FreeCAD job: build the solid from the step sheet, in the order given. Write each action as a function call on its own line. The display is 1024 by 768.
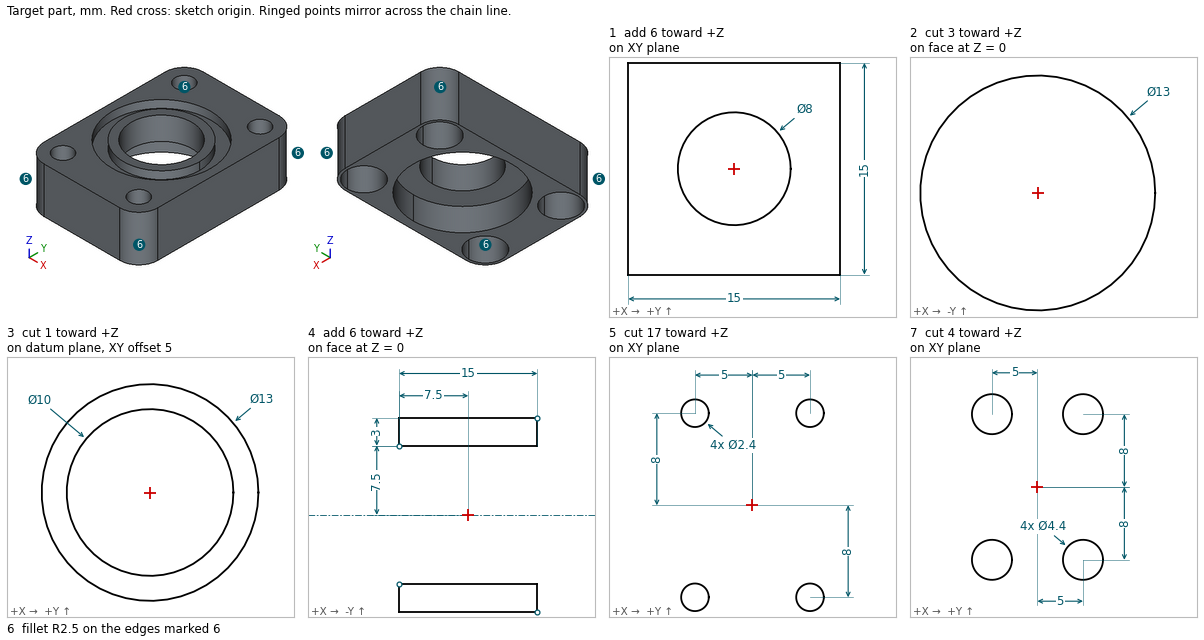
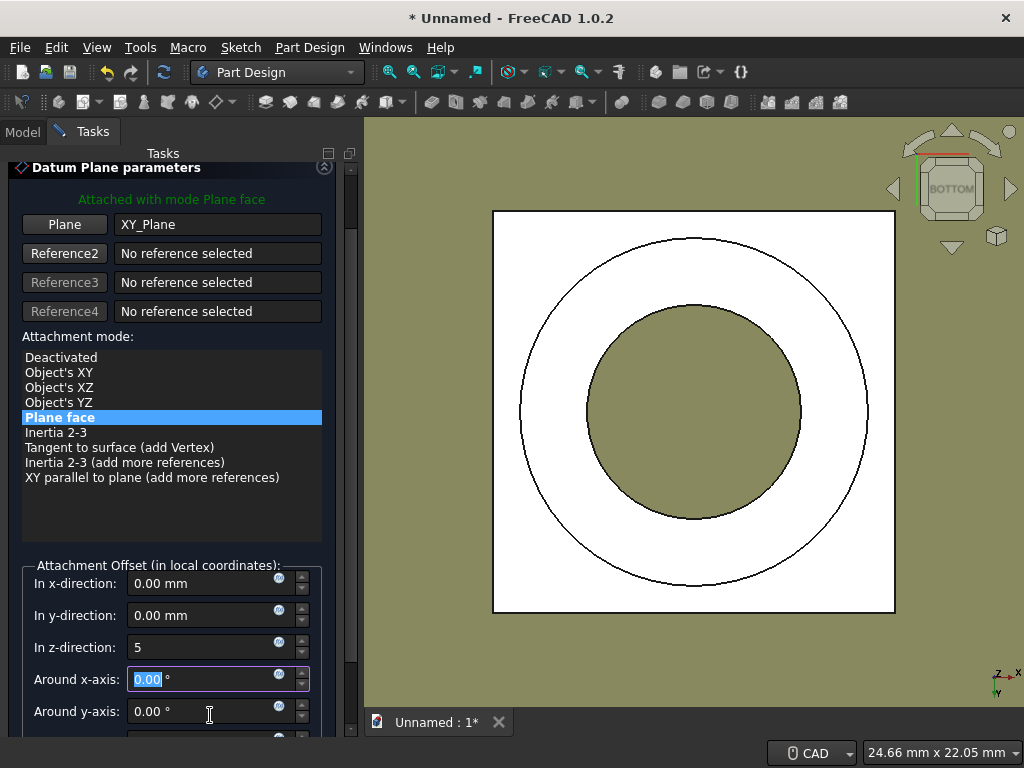
scroll(351, 450, up, 2)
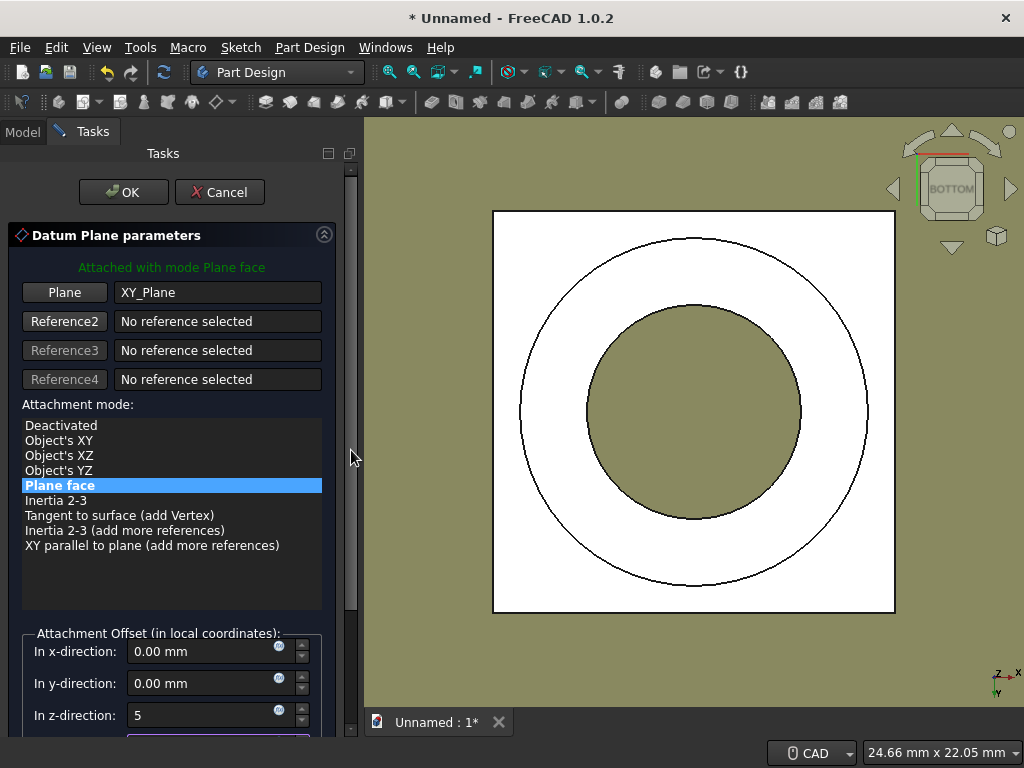
click(124, 192)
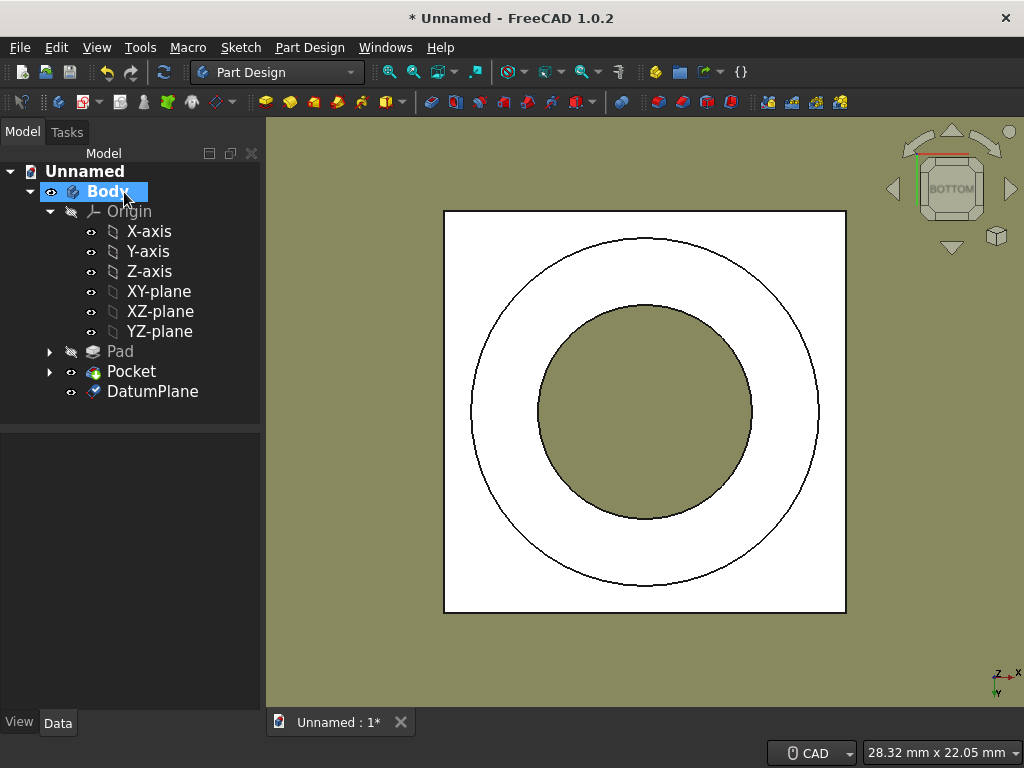
click(116, 392)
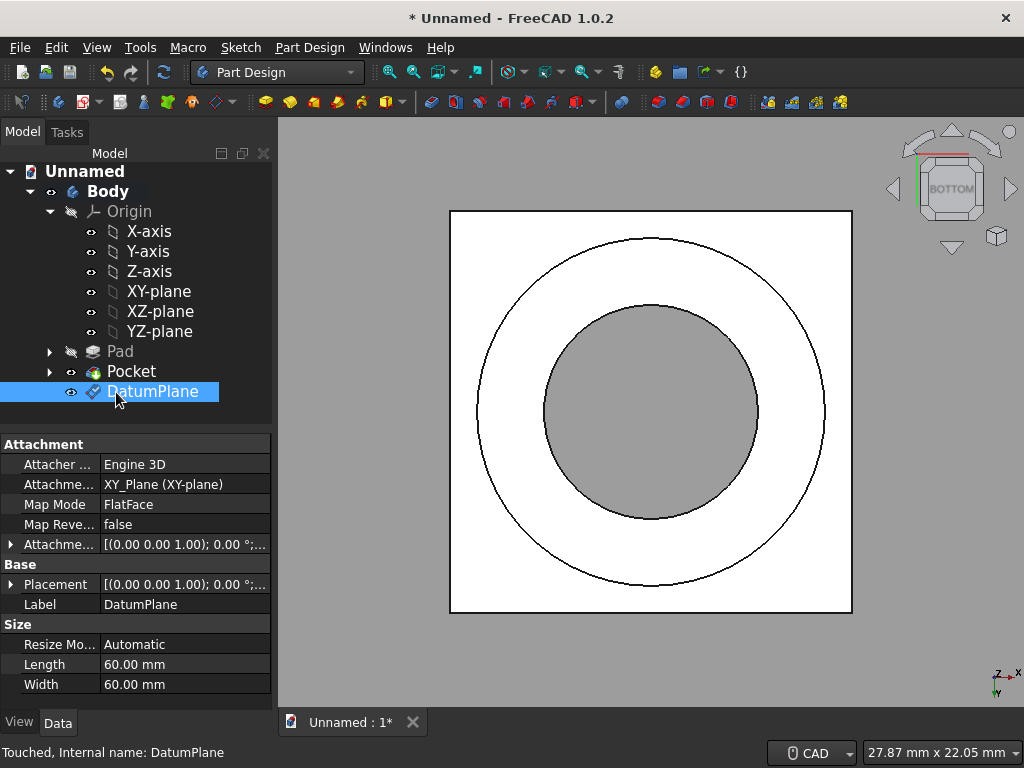
click(84, 102)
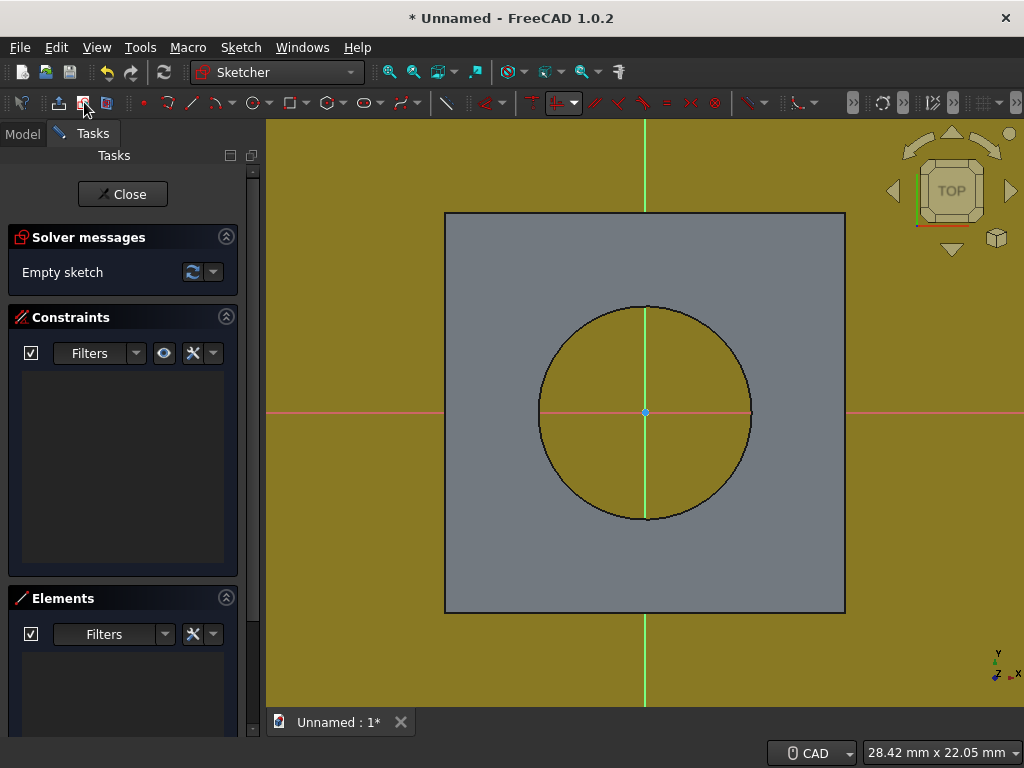
key(q)
key(s)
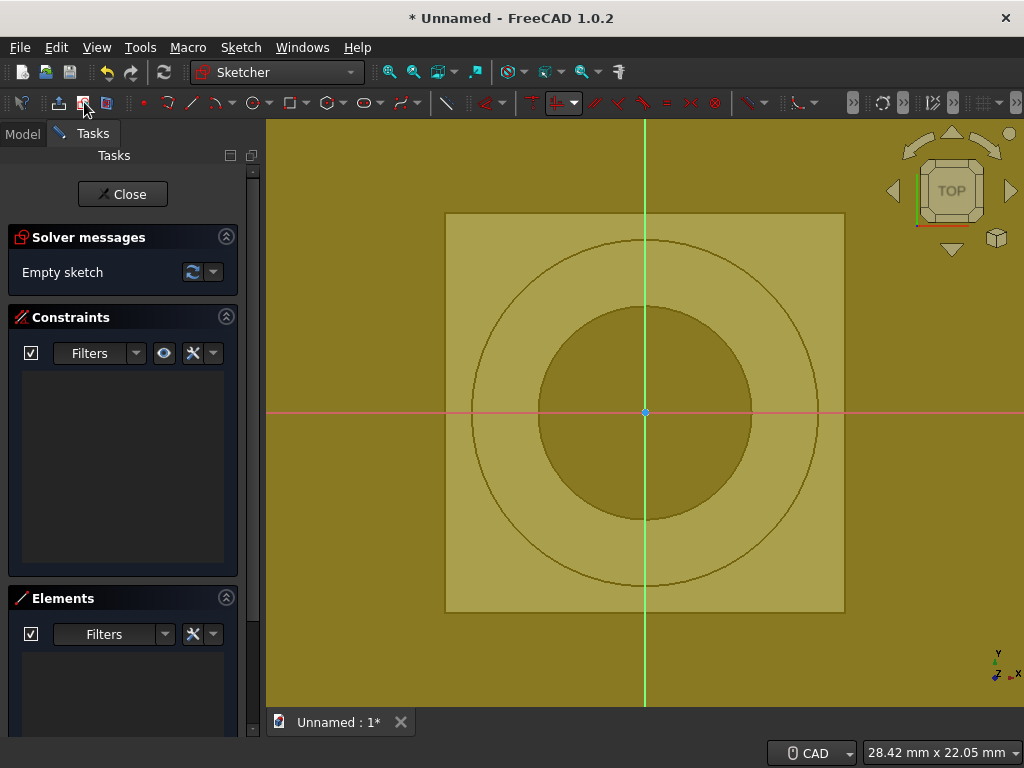
click(254, 104)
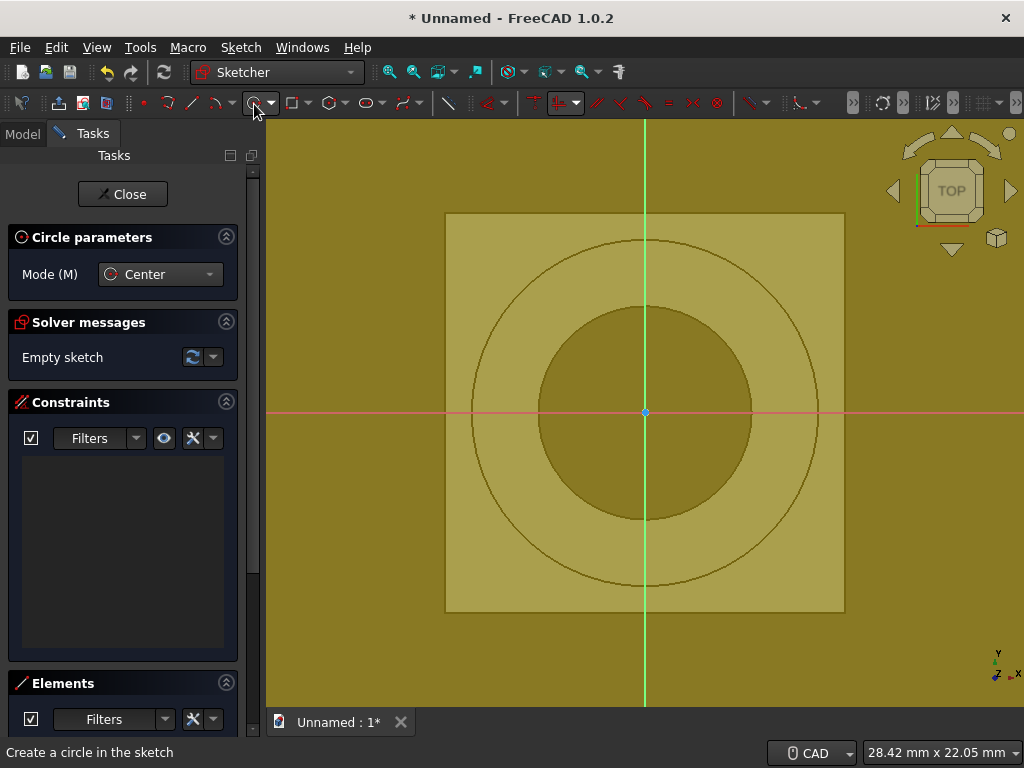
click(645, 413)
click(768, 290)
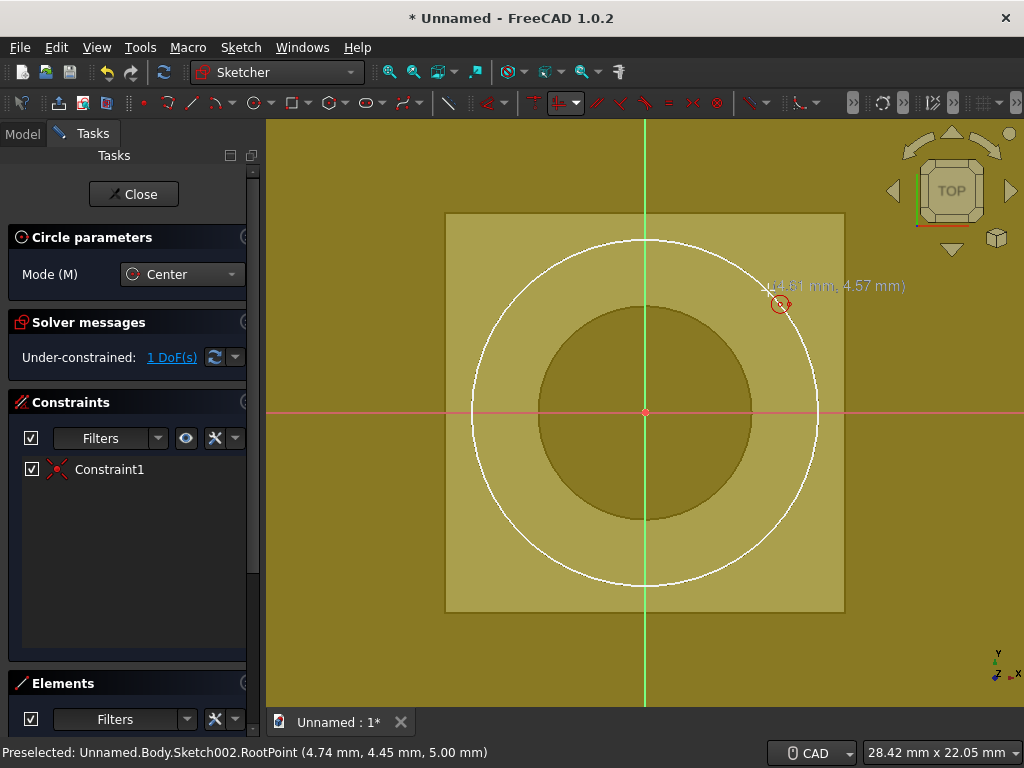
click(645, 413)
click(739, 319)
key(Escape)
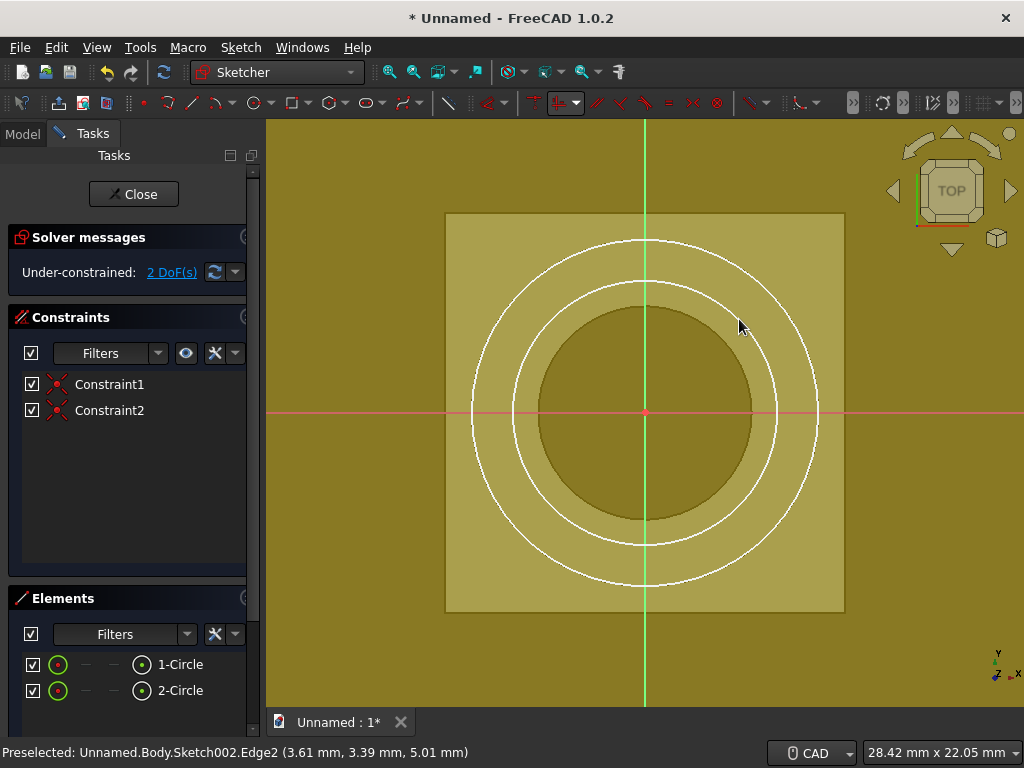
click(488, 104)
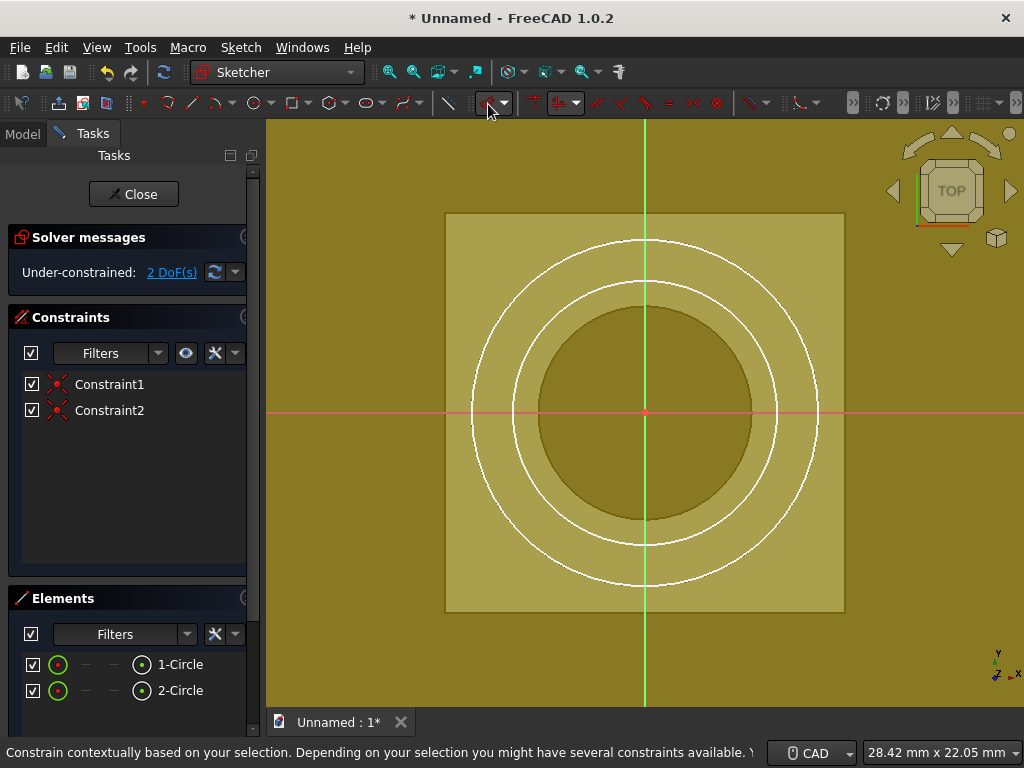
click(767, 290)
click(790, 267)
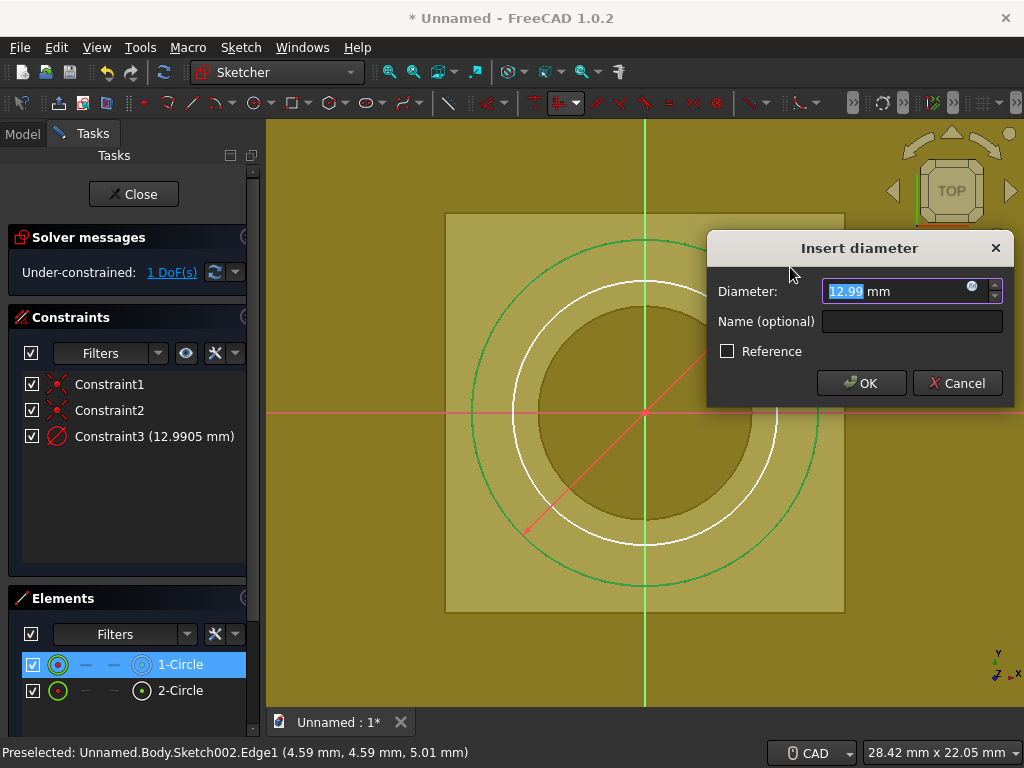
text(13)
key(Return)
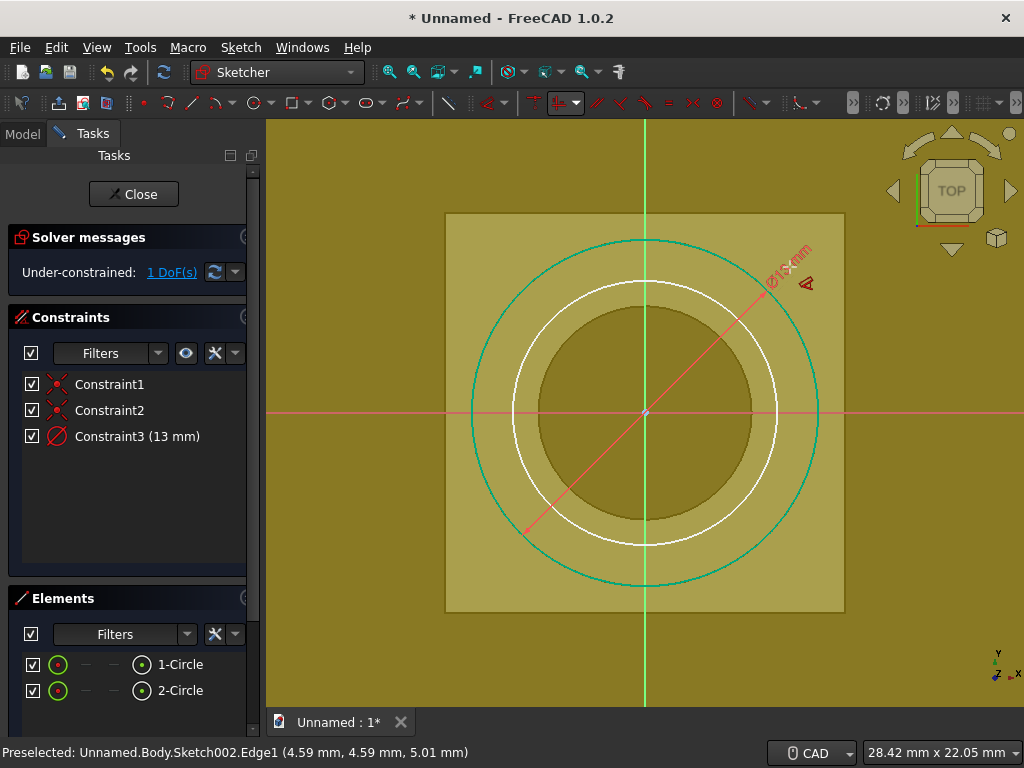
click(738, 319)
click(824, 359)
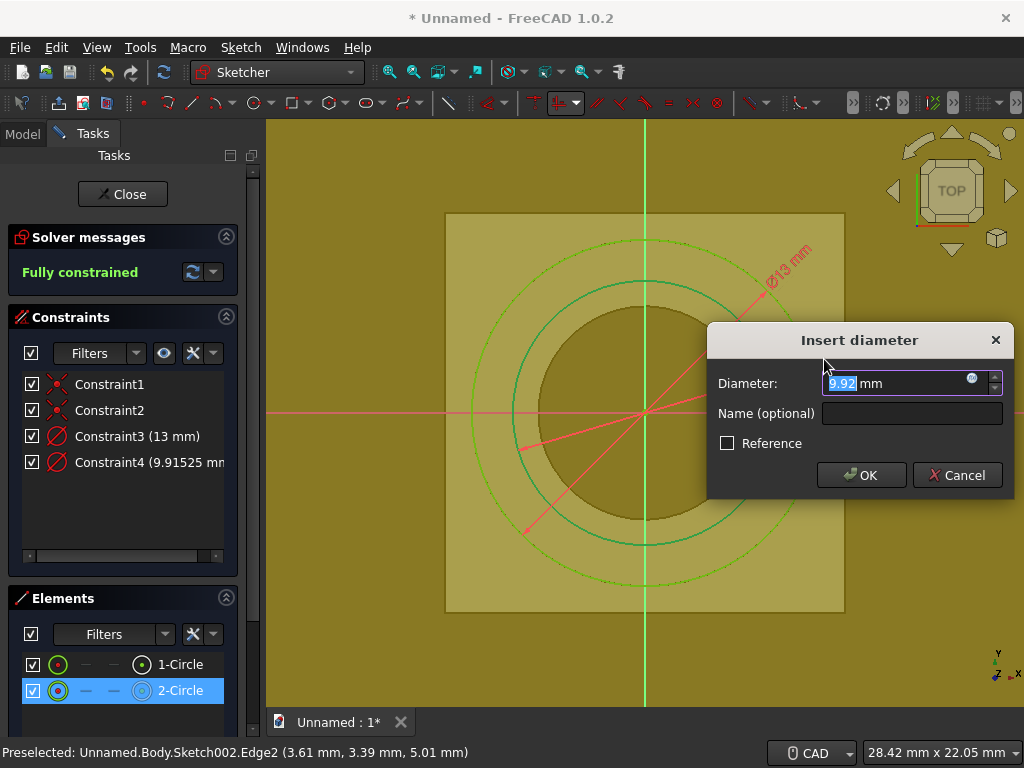
text(10)
key(Return)
key(Escape)